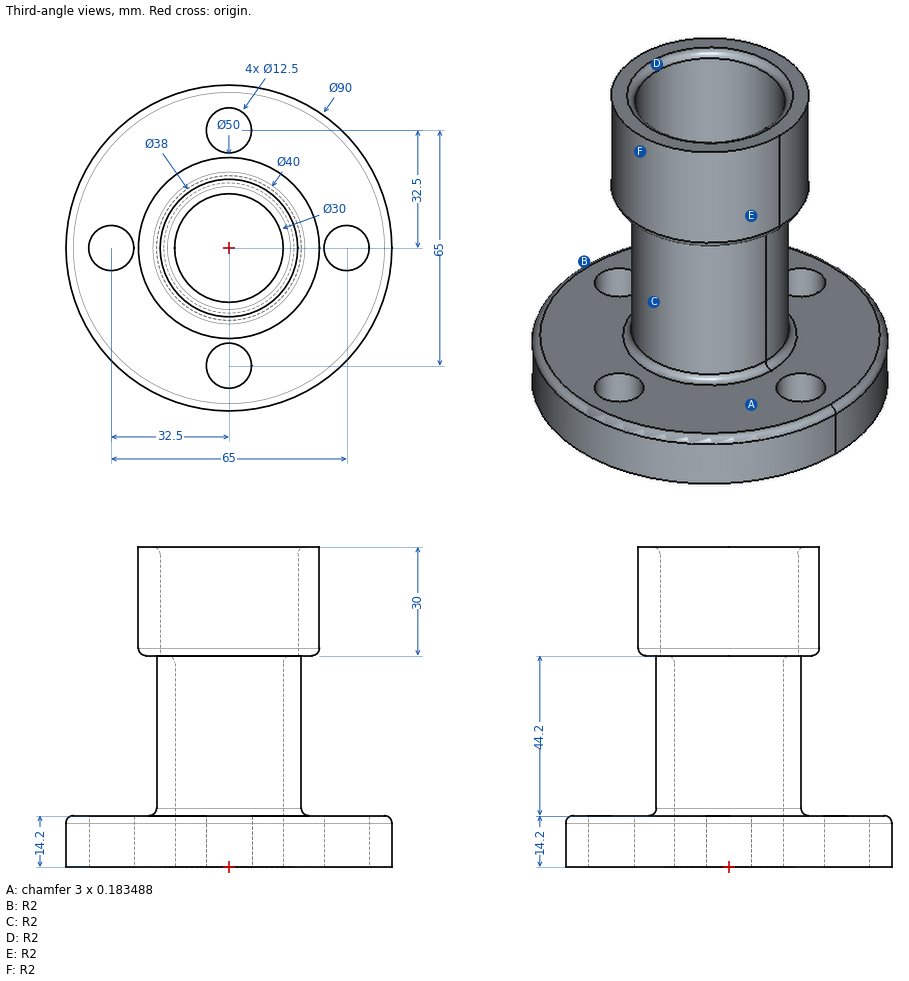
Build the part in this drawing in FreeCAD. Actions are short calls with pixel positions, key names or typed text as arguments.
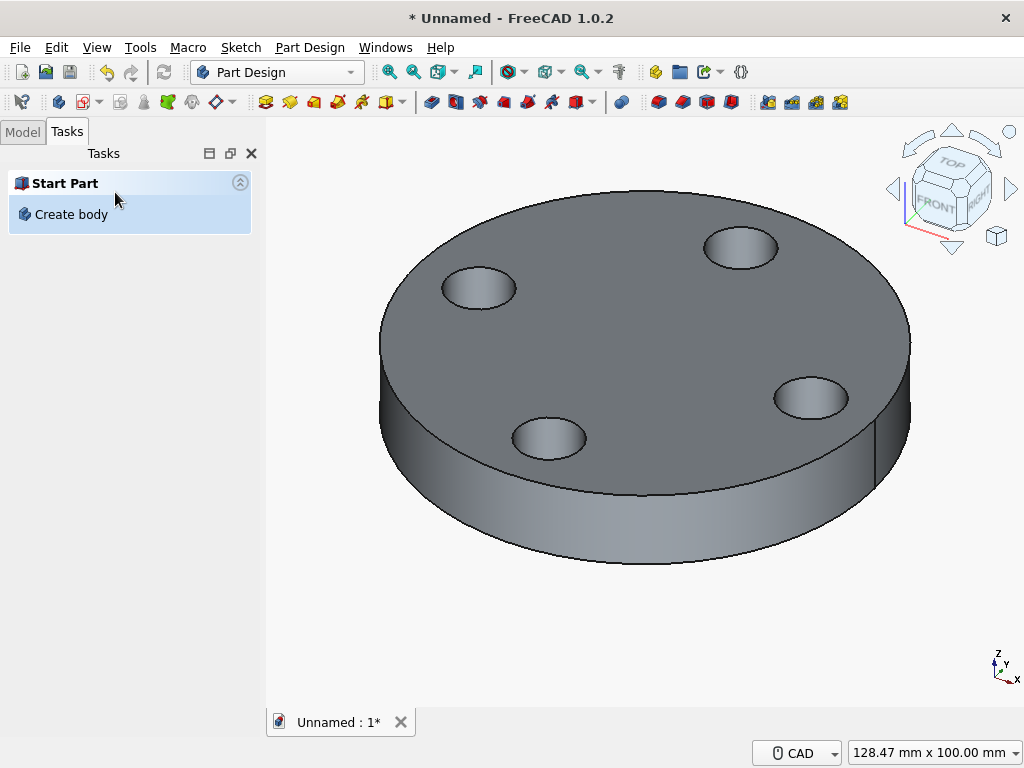
click(645, 342)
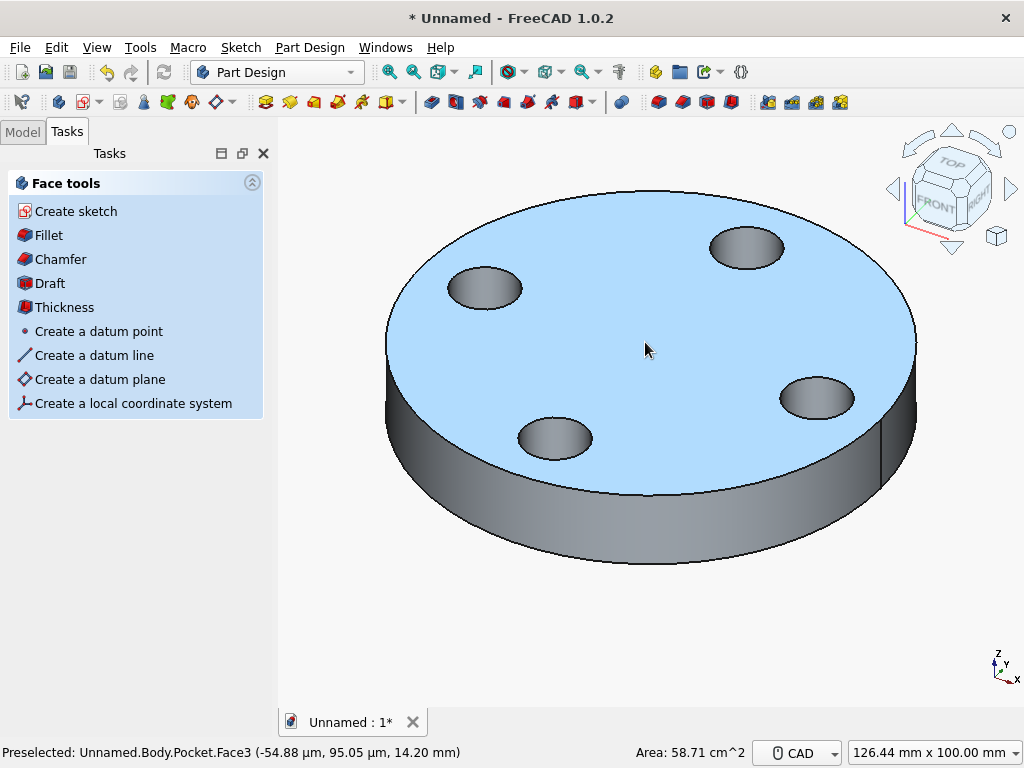
click(84, 102)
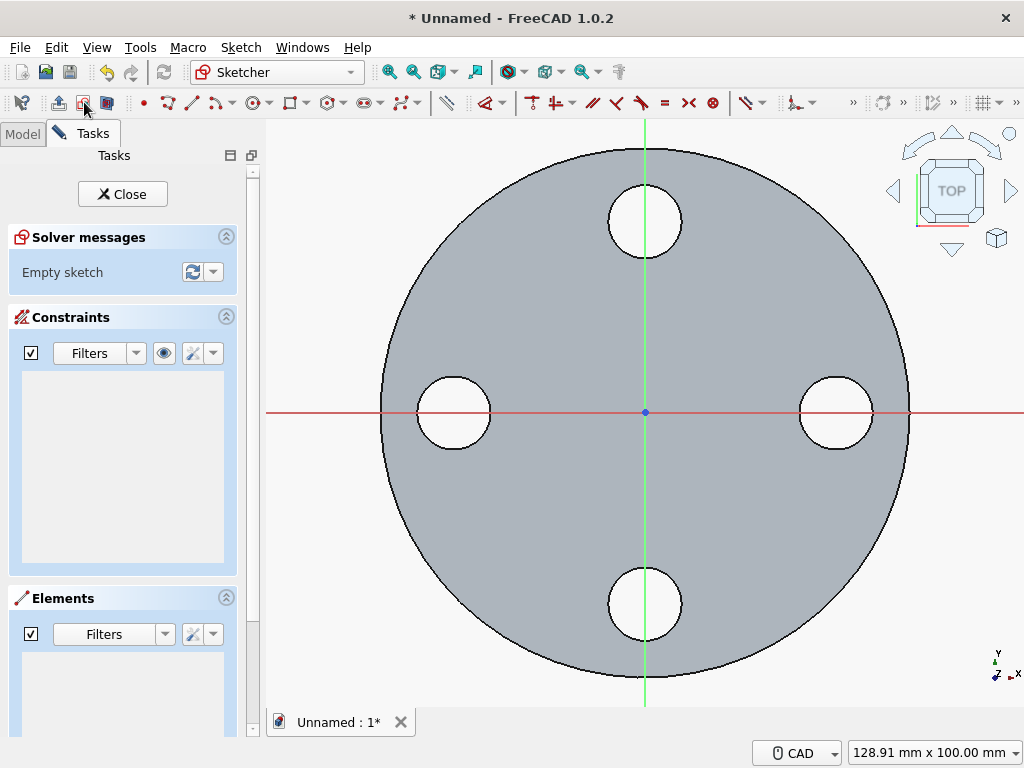
scroll(784, 413, up, 2)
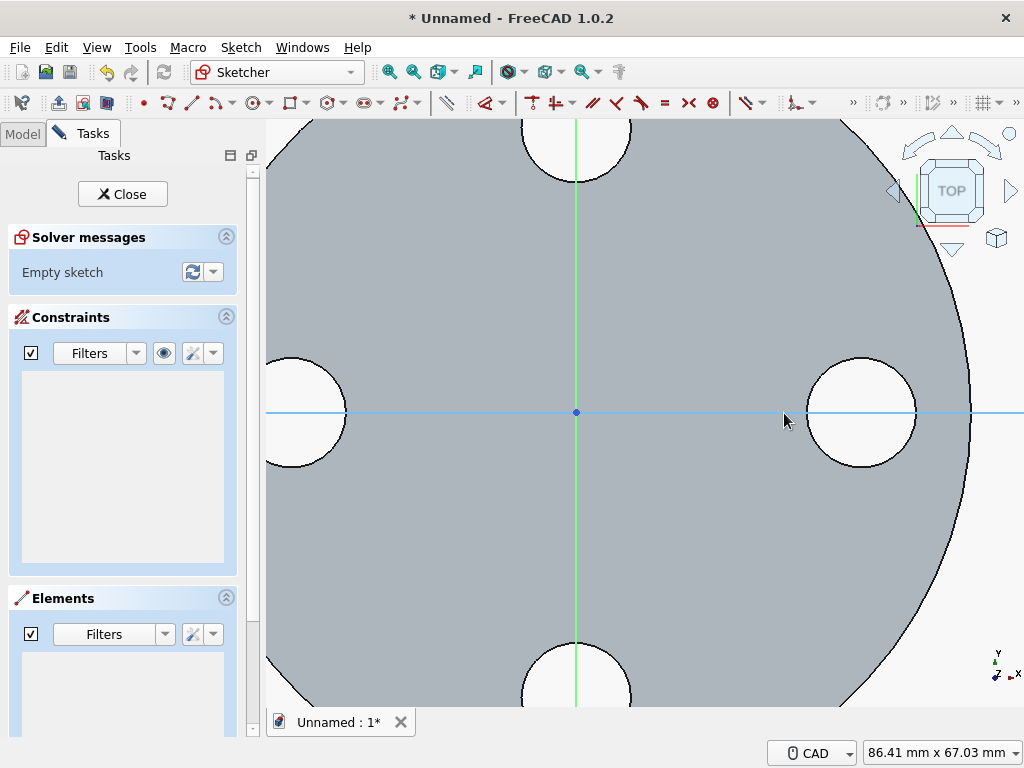
click(254, 104)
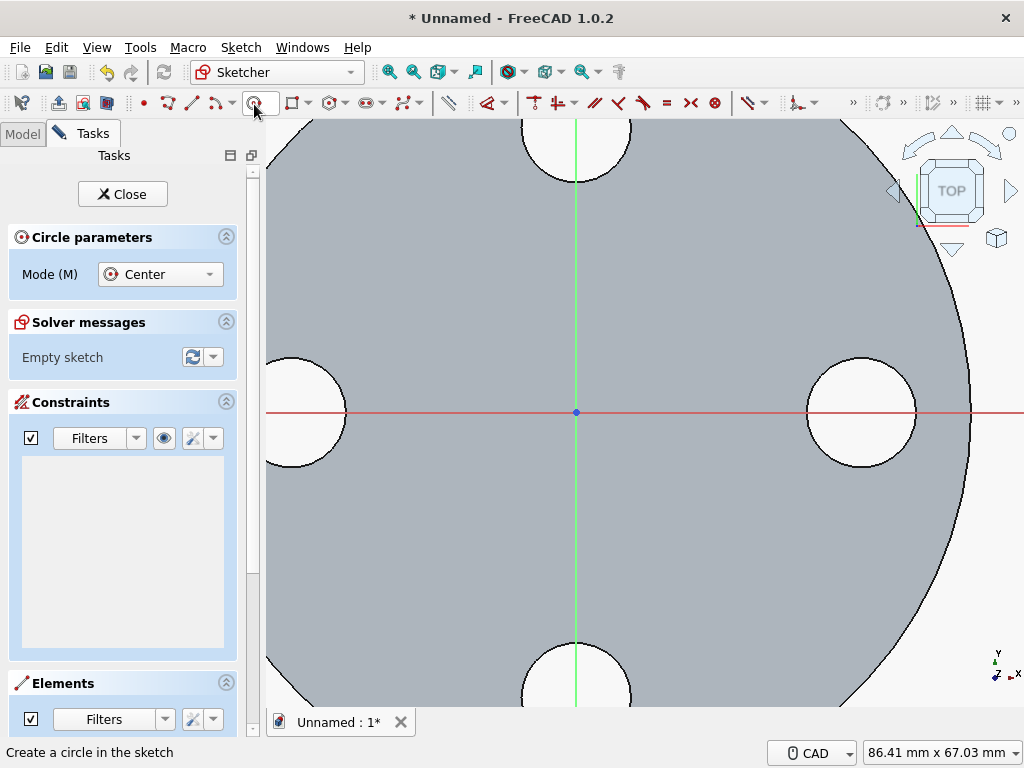
click(576, 413)
move(700, 289)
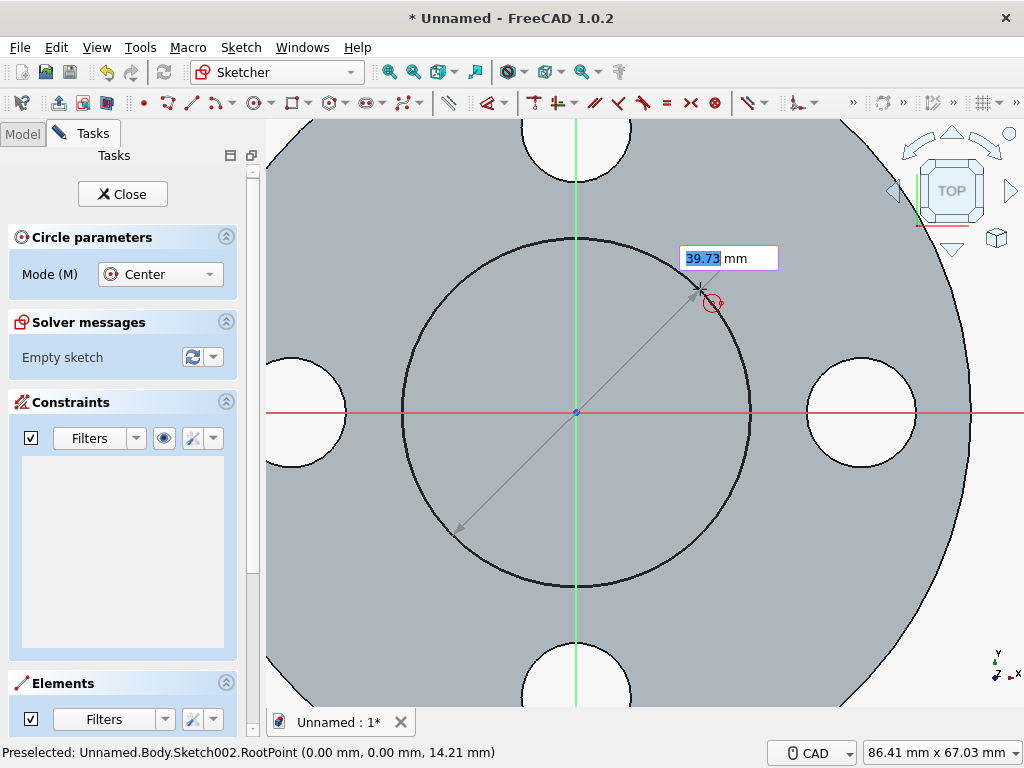
text(40)
key(Return)
key(Escape)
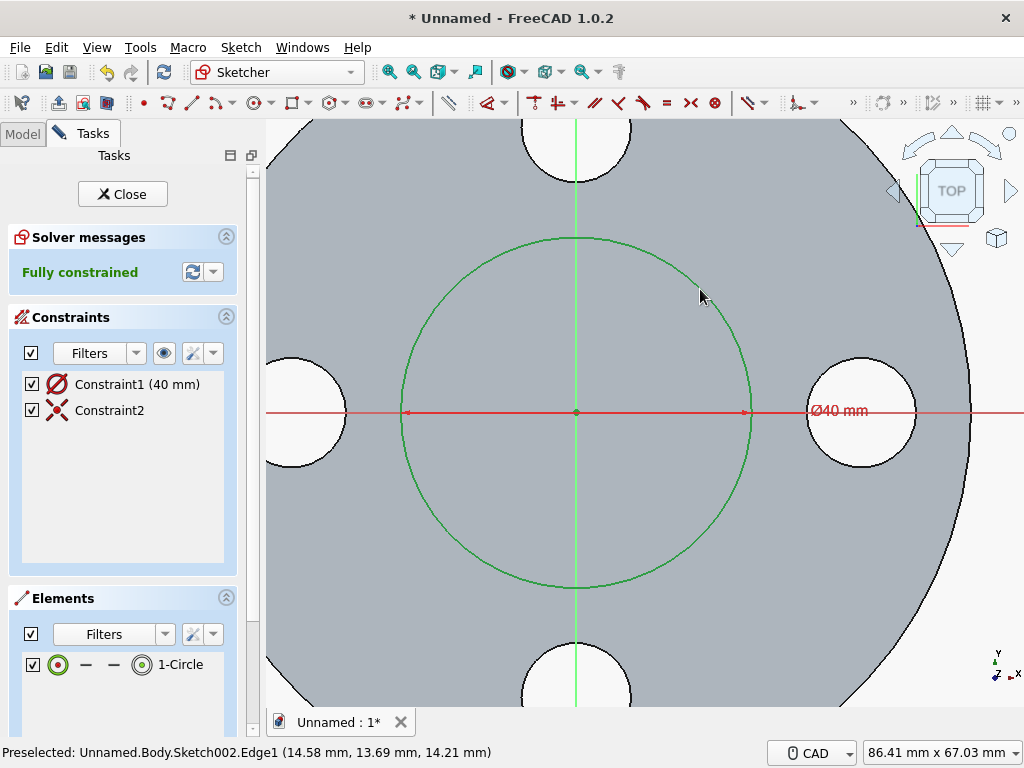
click(123, 194)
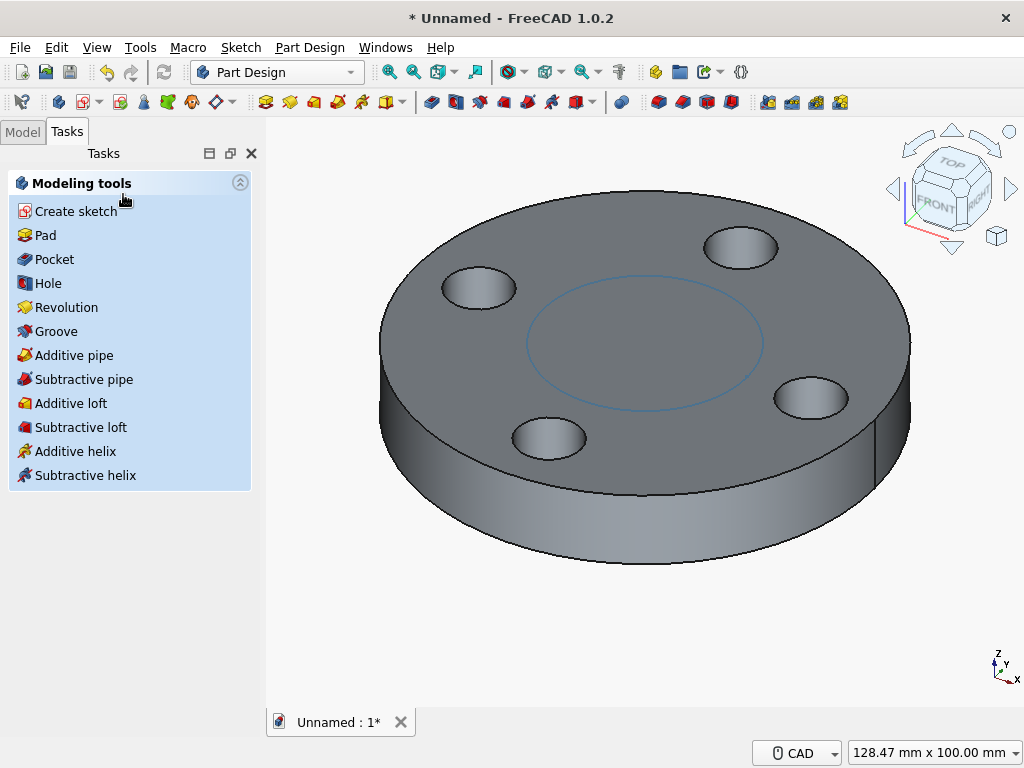
click(266, 102)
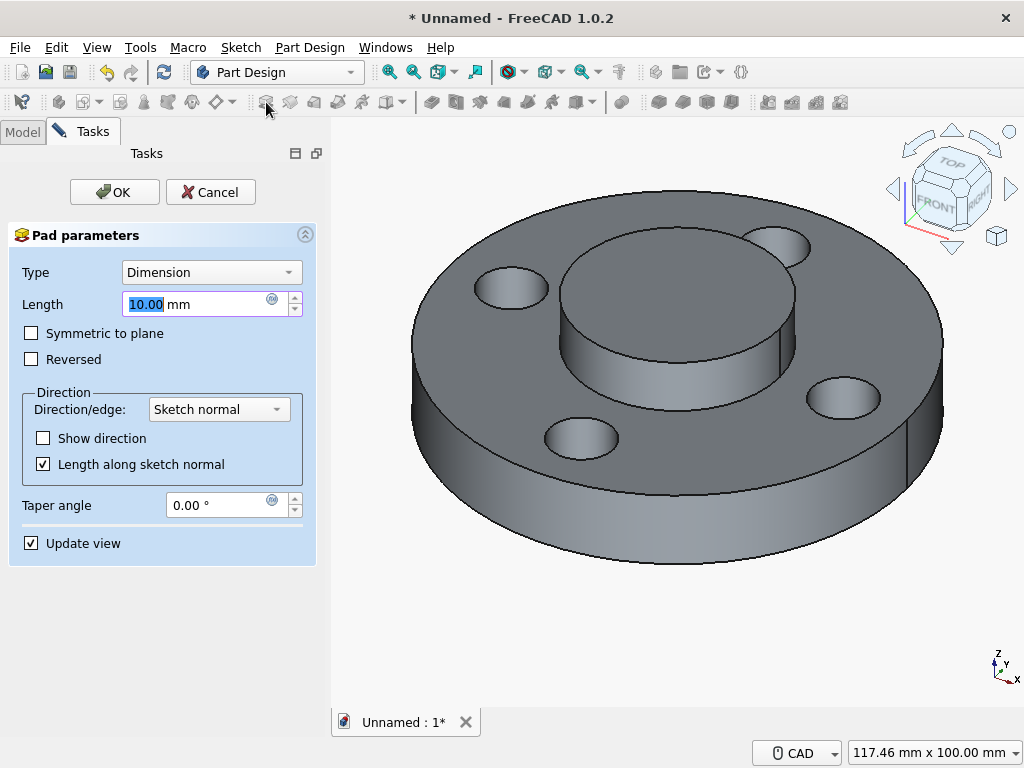
text(44.2)
key(Tab)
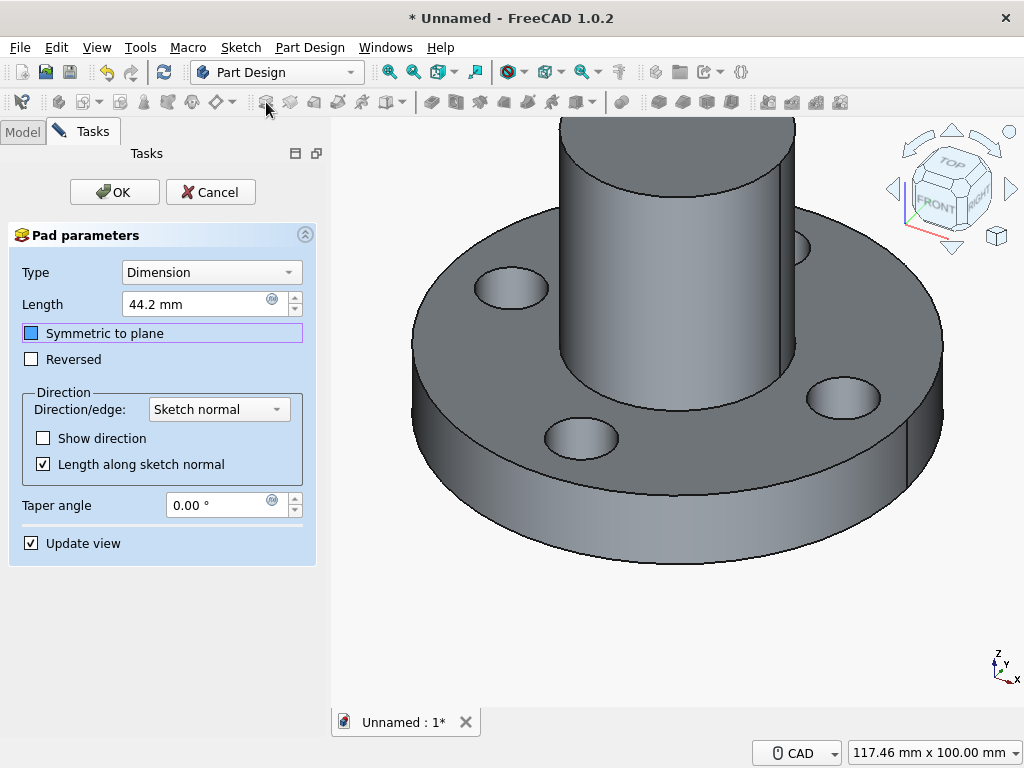
click(115, 192)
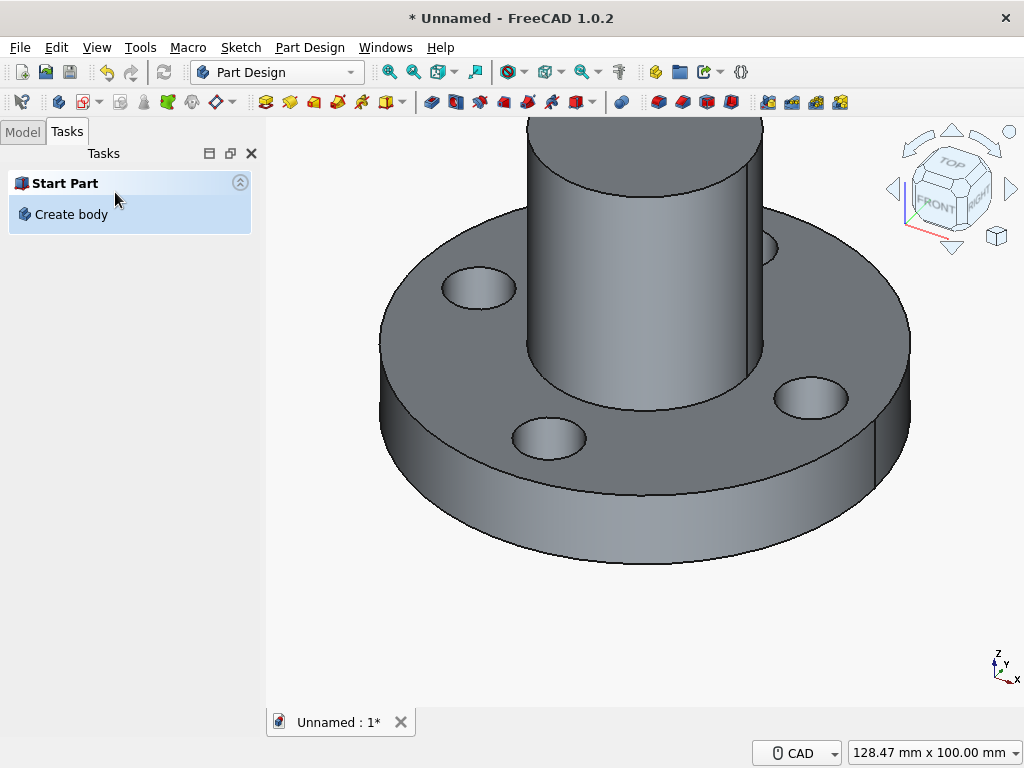
key(v)
key(f)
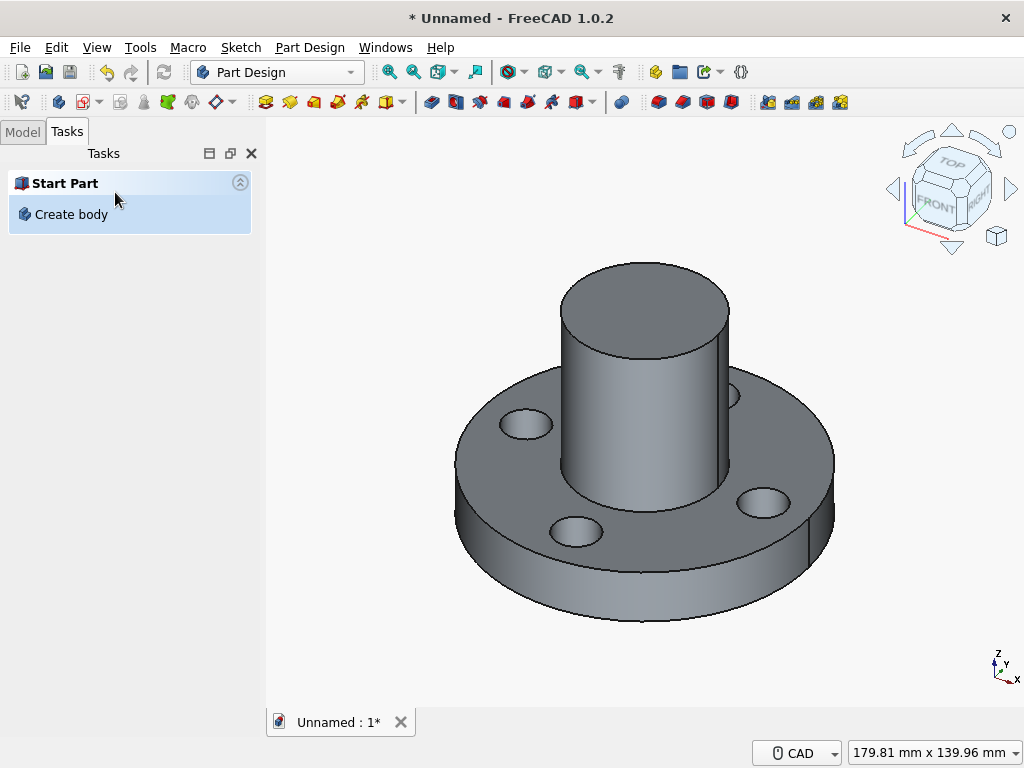
click(84, 102)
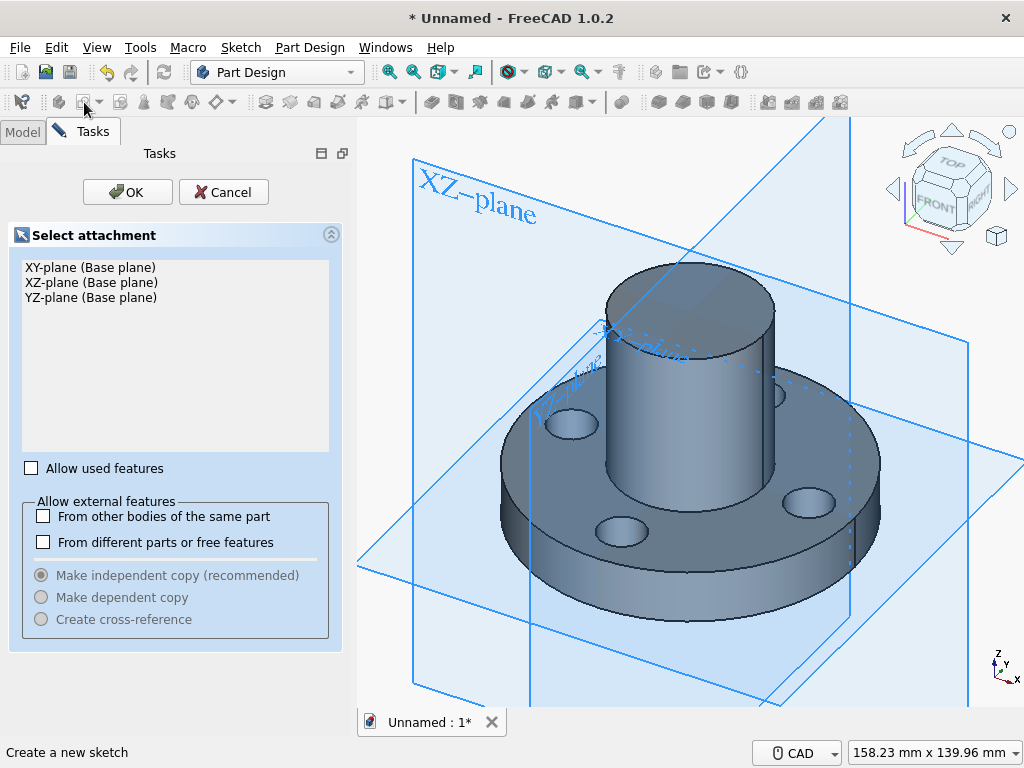
click(82, 268)